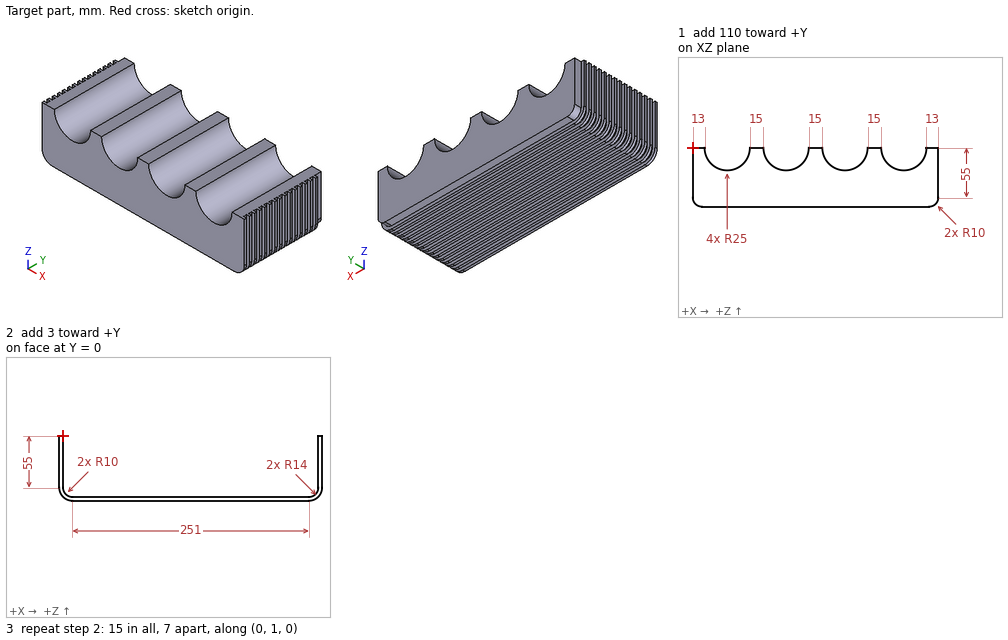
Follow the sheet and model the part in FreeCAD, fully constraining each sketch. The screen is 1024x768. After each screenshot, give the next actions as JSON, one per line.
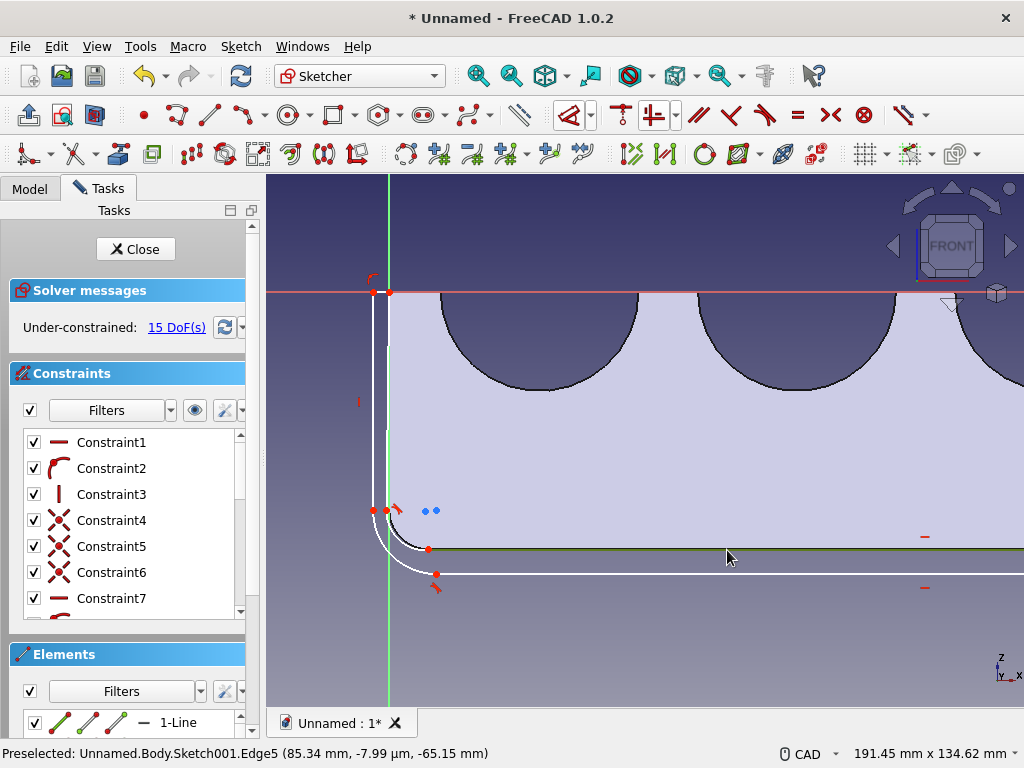
{"action": "left_click", "coordinate": [391, 529]}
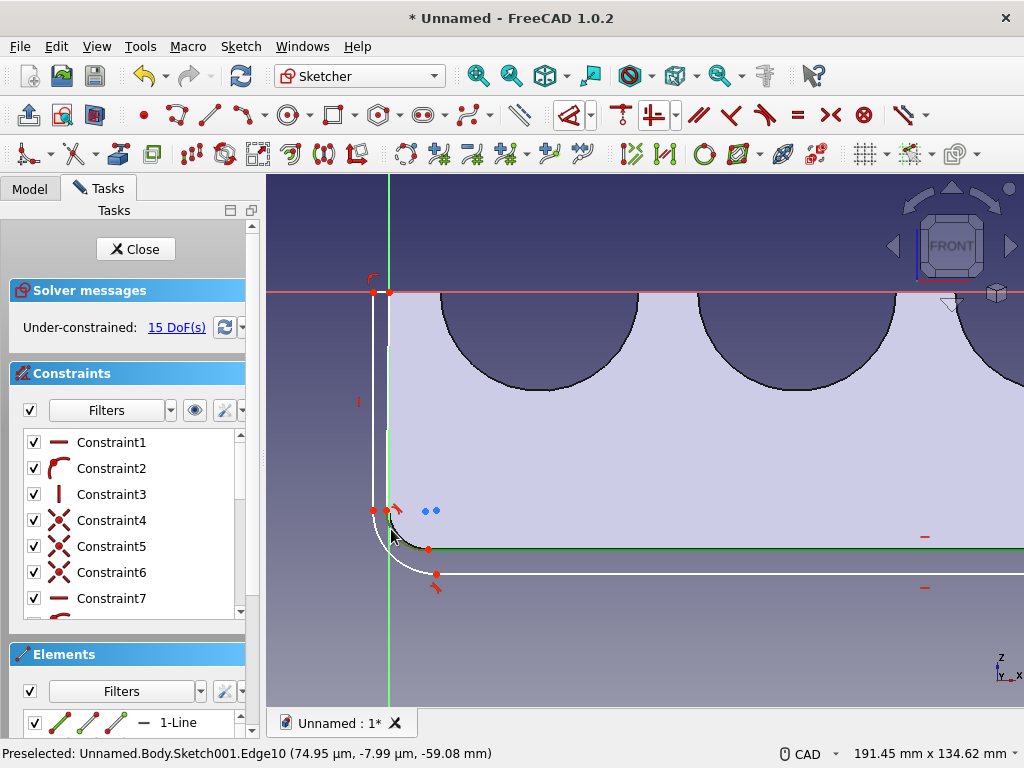
{"action": "left_click", "coordinate": [765, 116]}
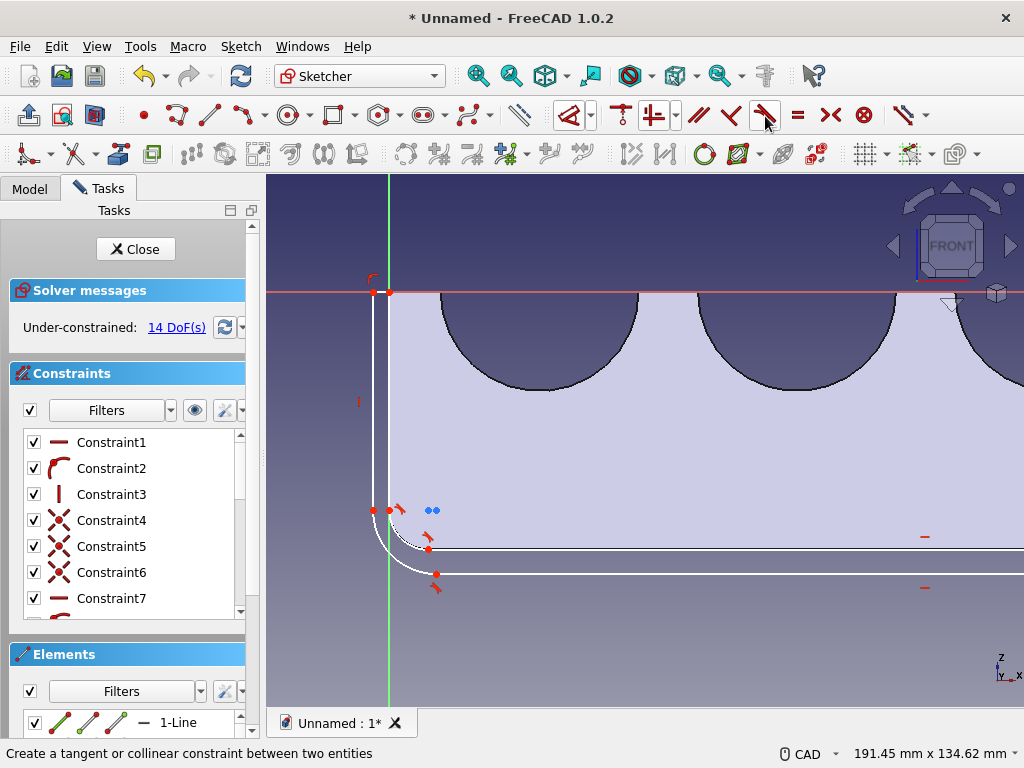
{"action": "left_click", "coordinate": [727, 550]}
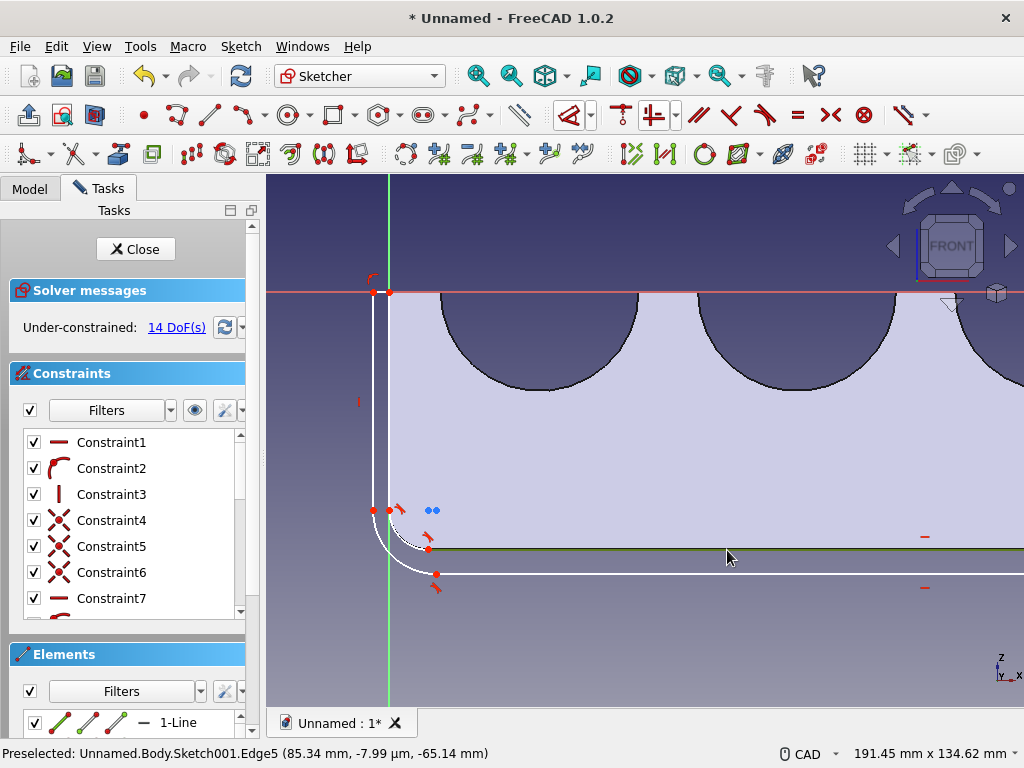
{"action": "scroll", "coordinate": [373, 447], "scroll_direction": "down", "scroll_amount": 5}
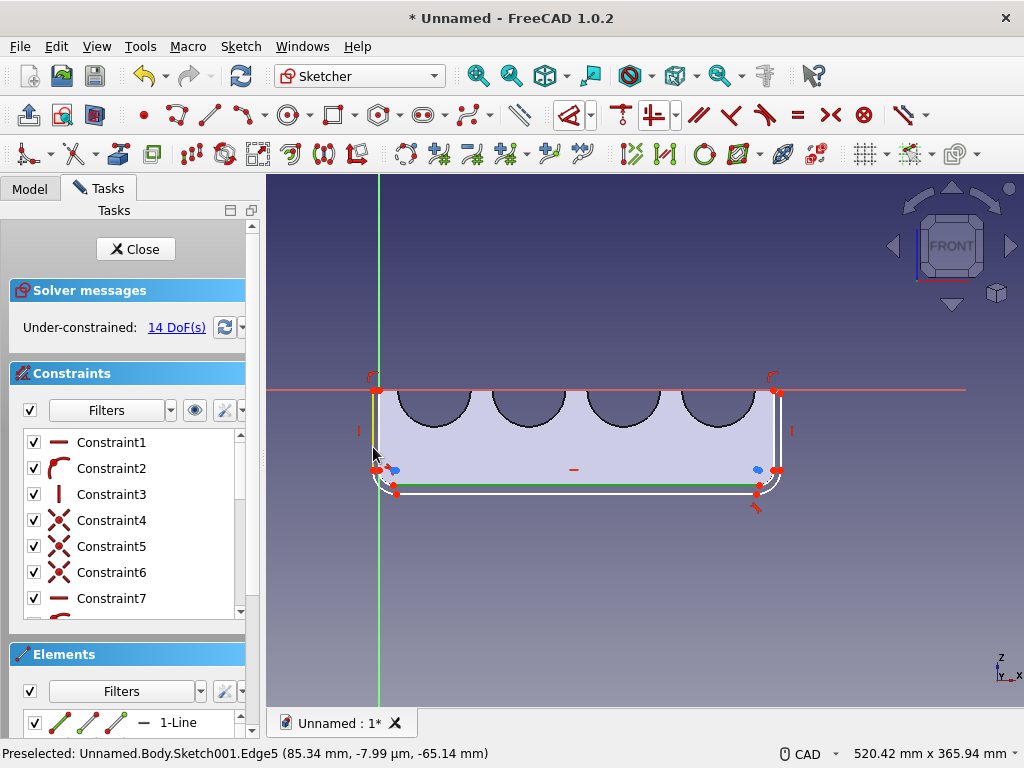
{"action": "scroll", "coordinate": [766, 484], "scroll_direction": "up", "scroll_amount": 4}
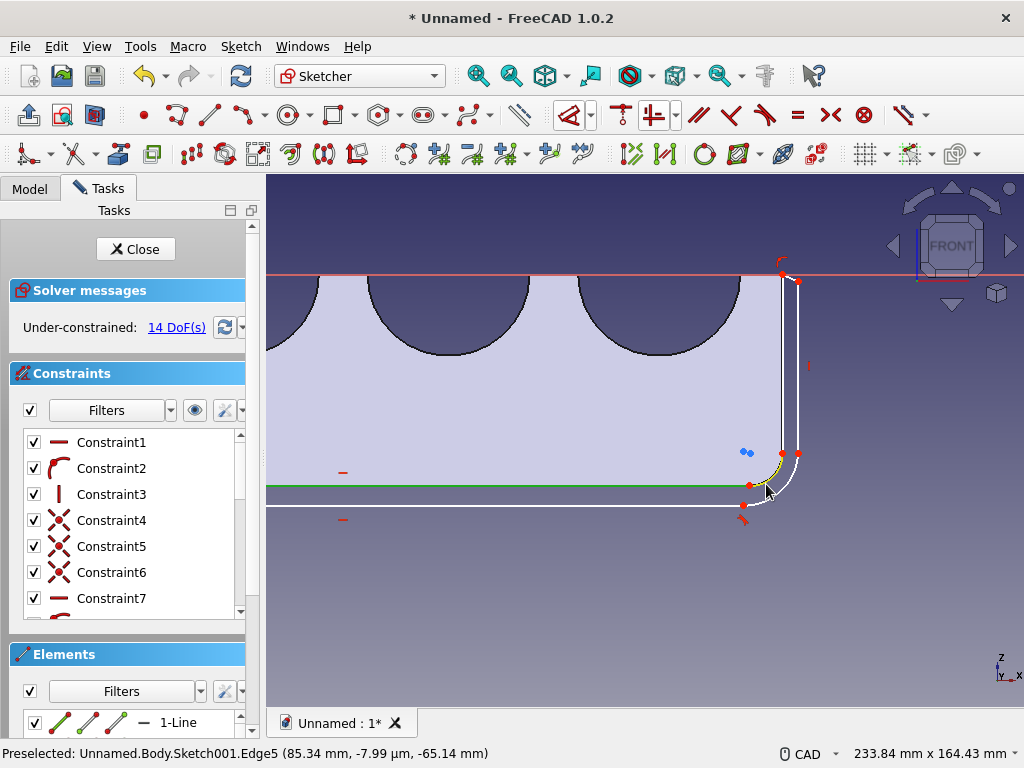
{"action": "left_click", "coordinate": [765, 483]}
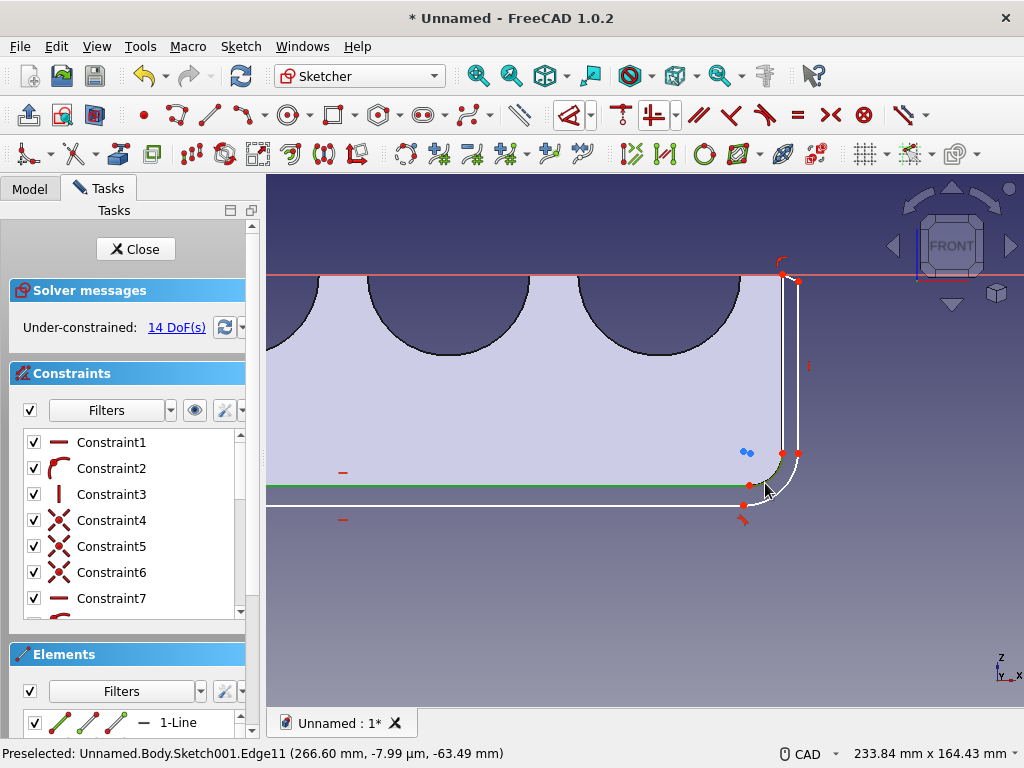
{"action": "left_click", "coordinate": [765, 116]}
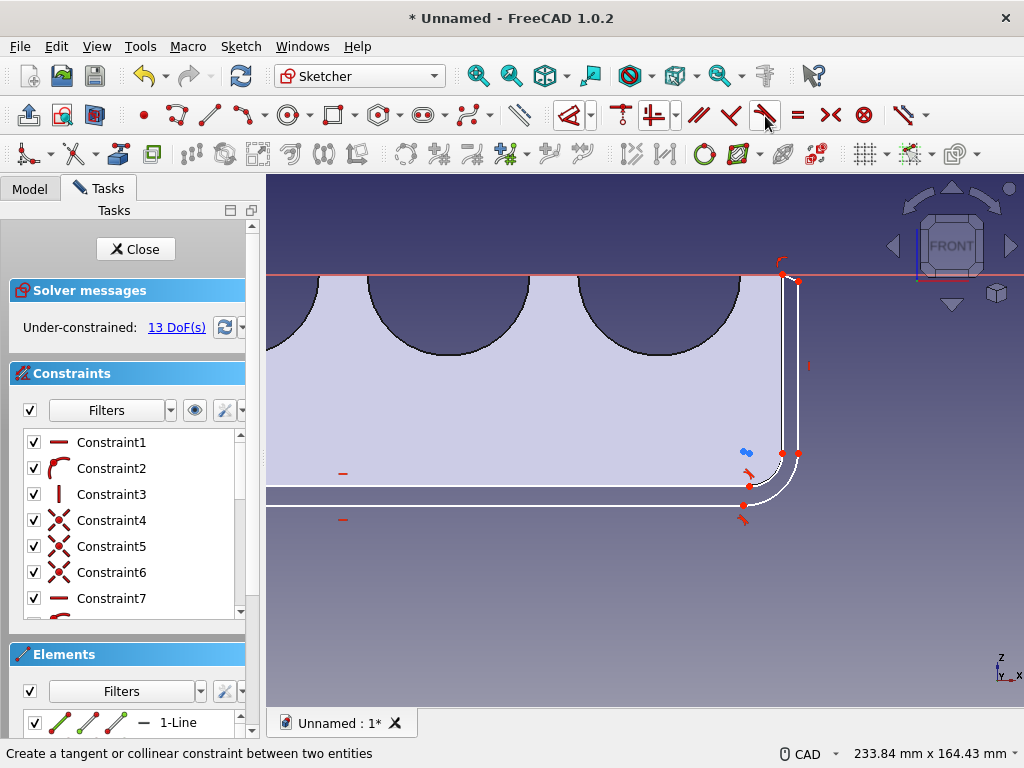
{"action": "left_click", "coordinate": [783, 400]}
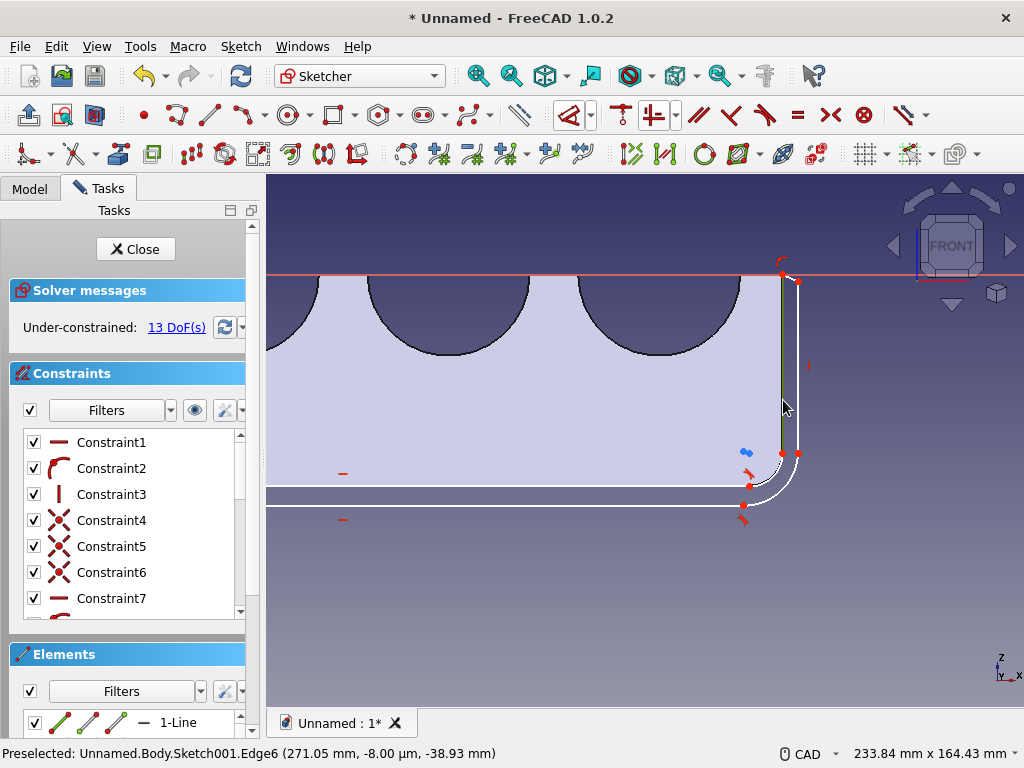
{"action": "left_click", "coordinate": [765, 483]}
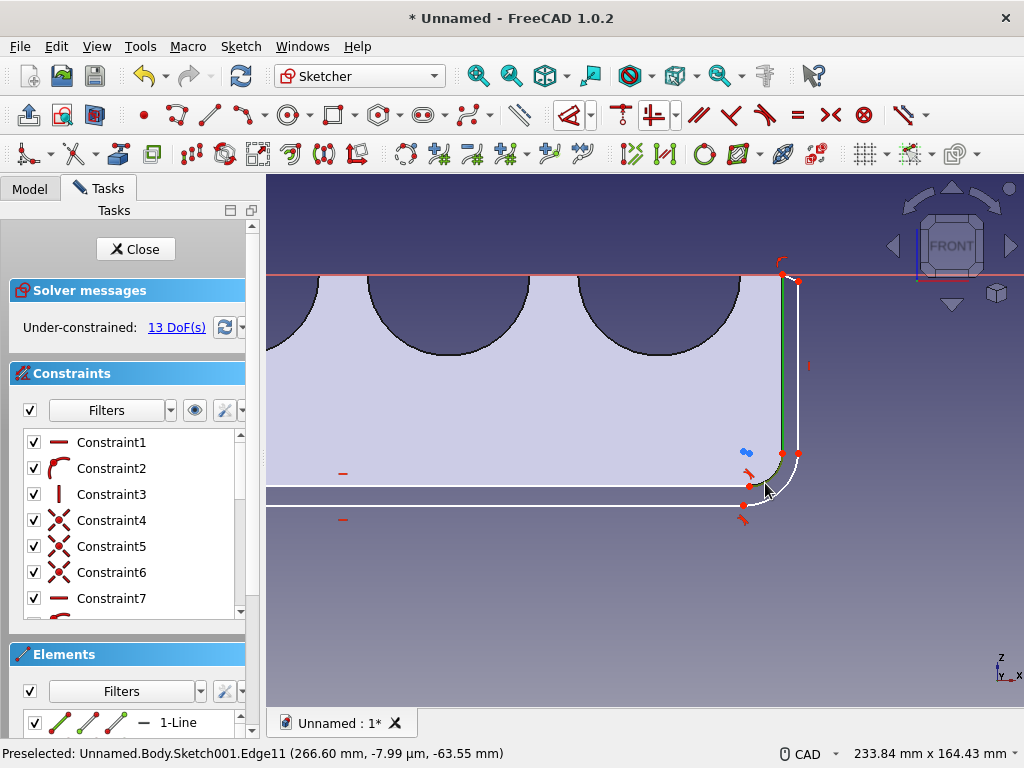
{"action": "key", "text": "t"}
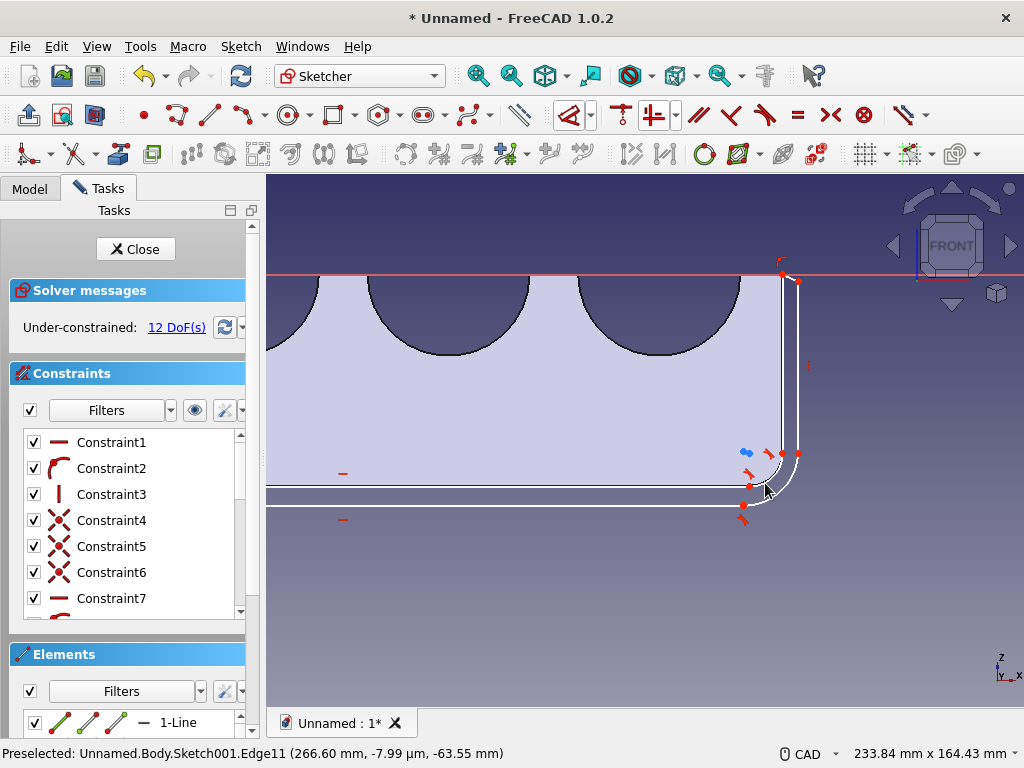
{"action": "left_click", "coordinate": [798, 333]}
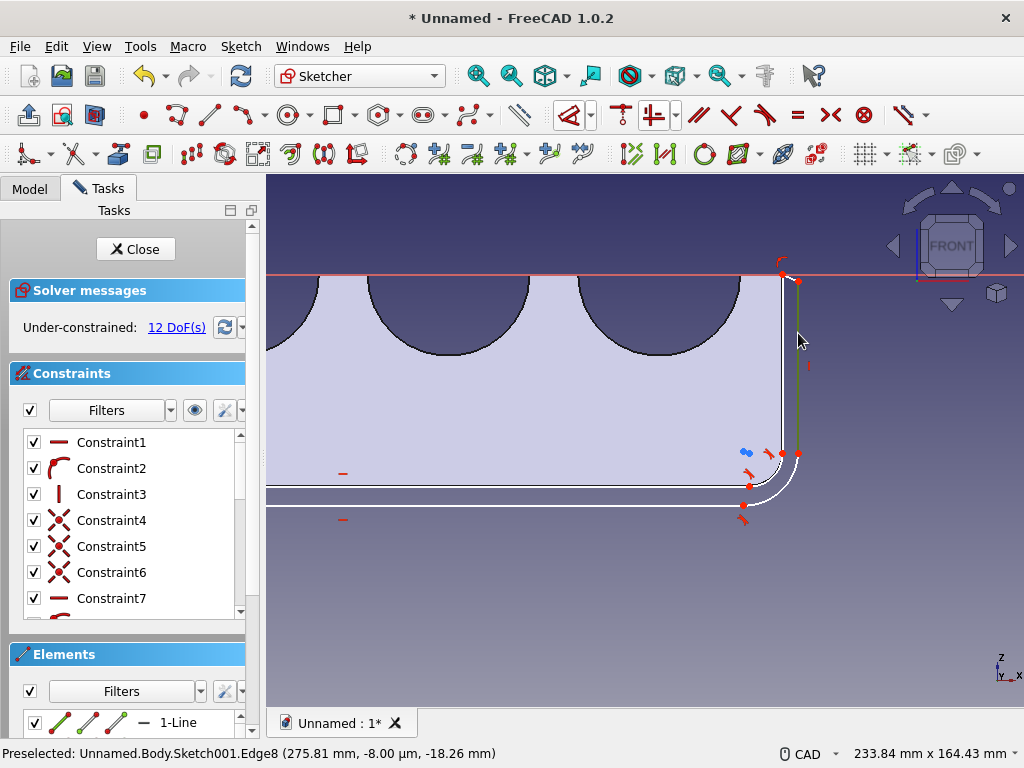
{"action": "left_click", "coordinate": [768, 500]}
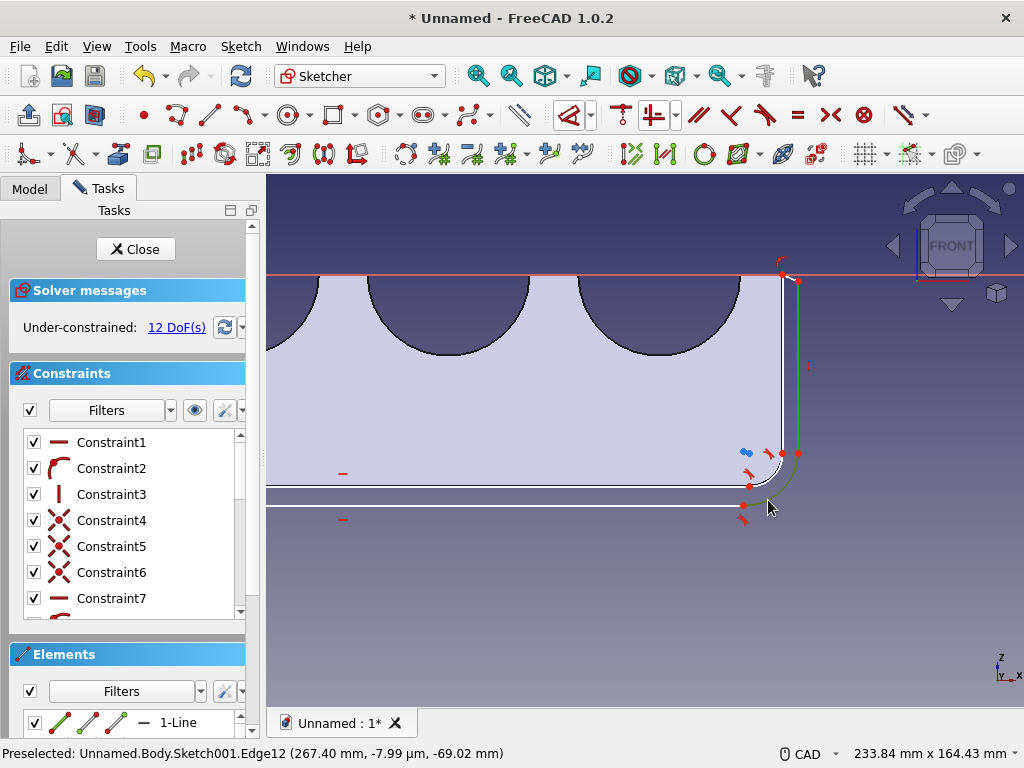
{"action": "left_click", "coordinate": [765, 116]}